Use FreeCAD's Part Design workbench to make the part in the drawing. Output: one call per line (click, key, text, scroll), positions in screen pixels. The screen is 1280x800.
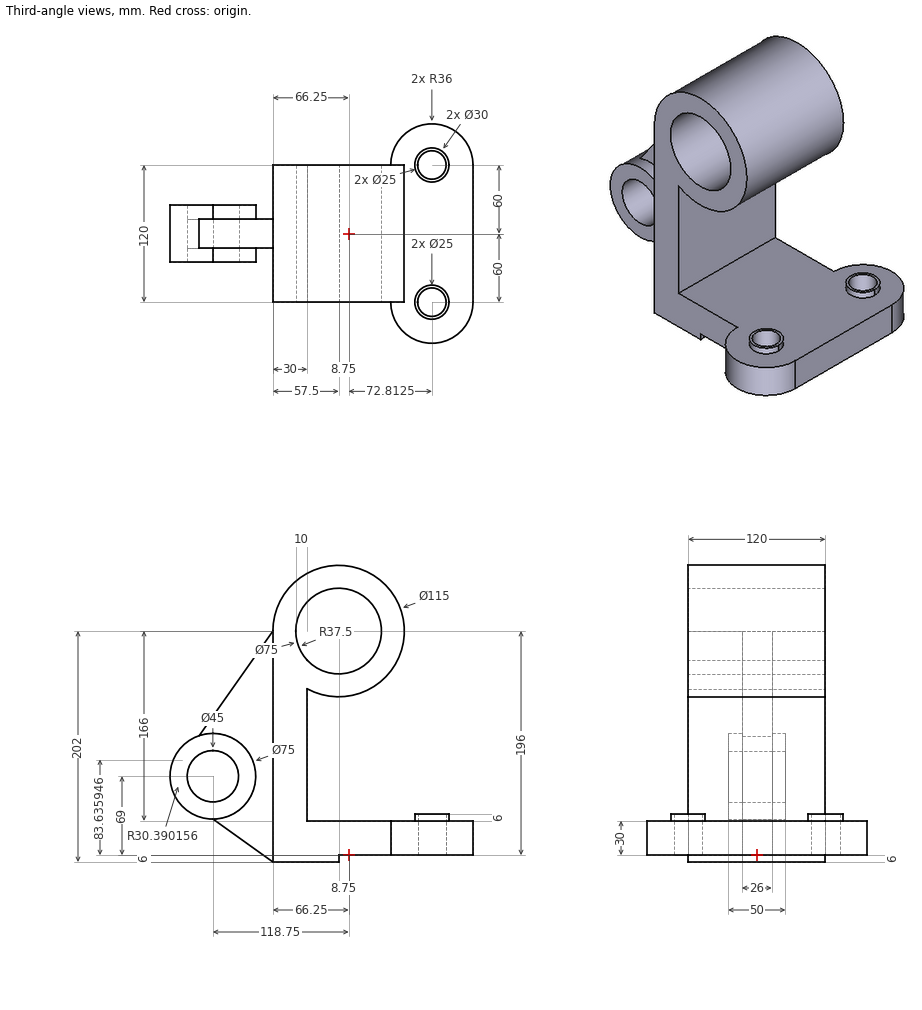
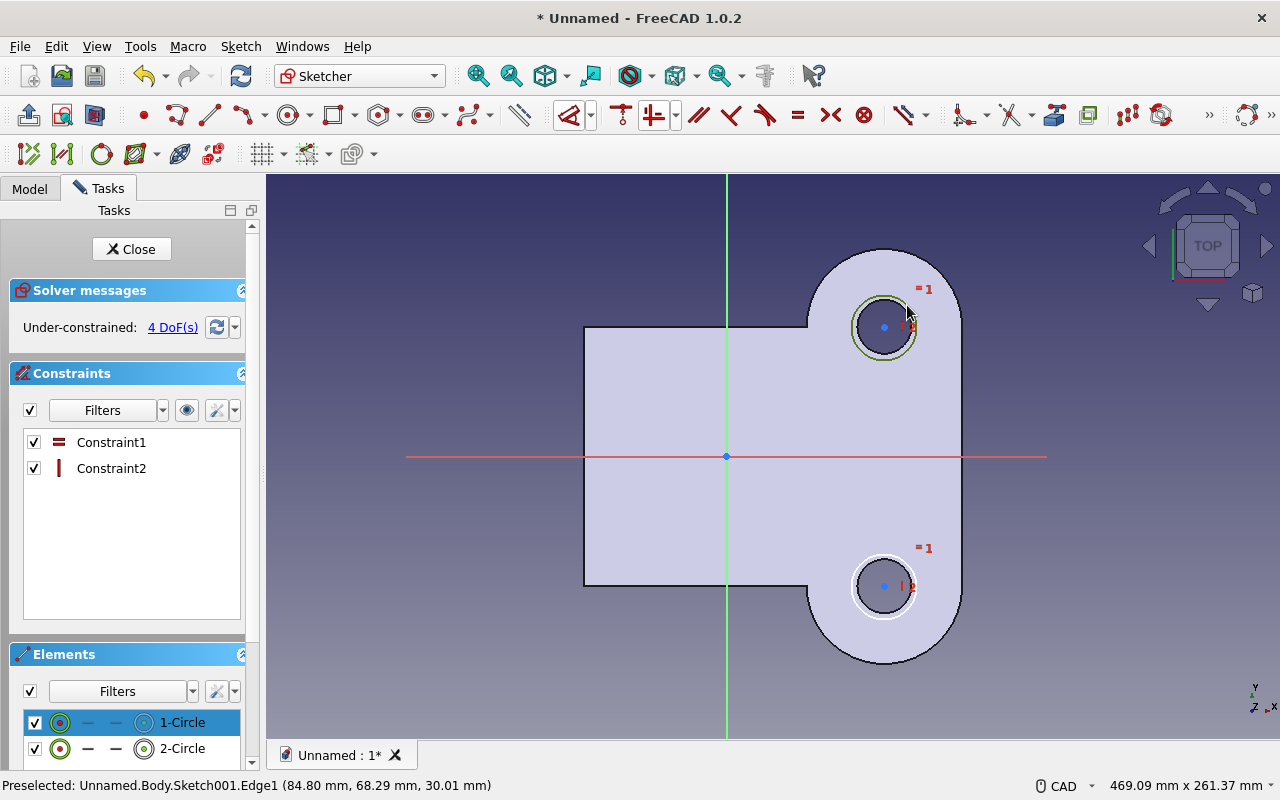
key(k)
key(o)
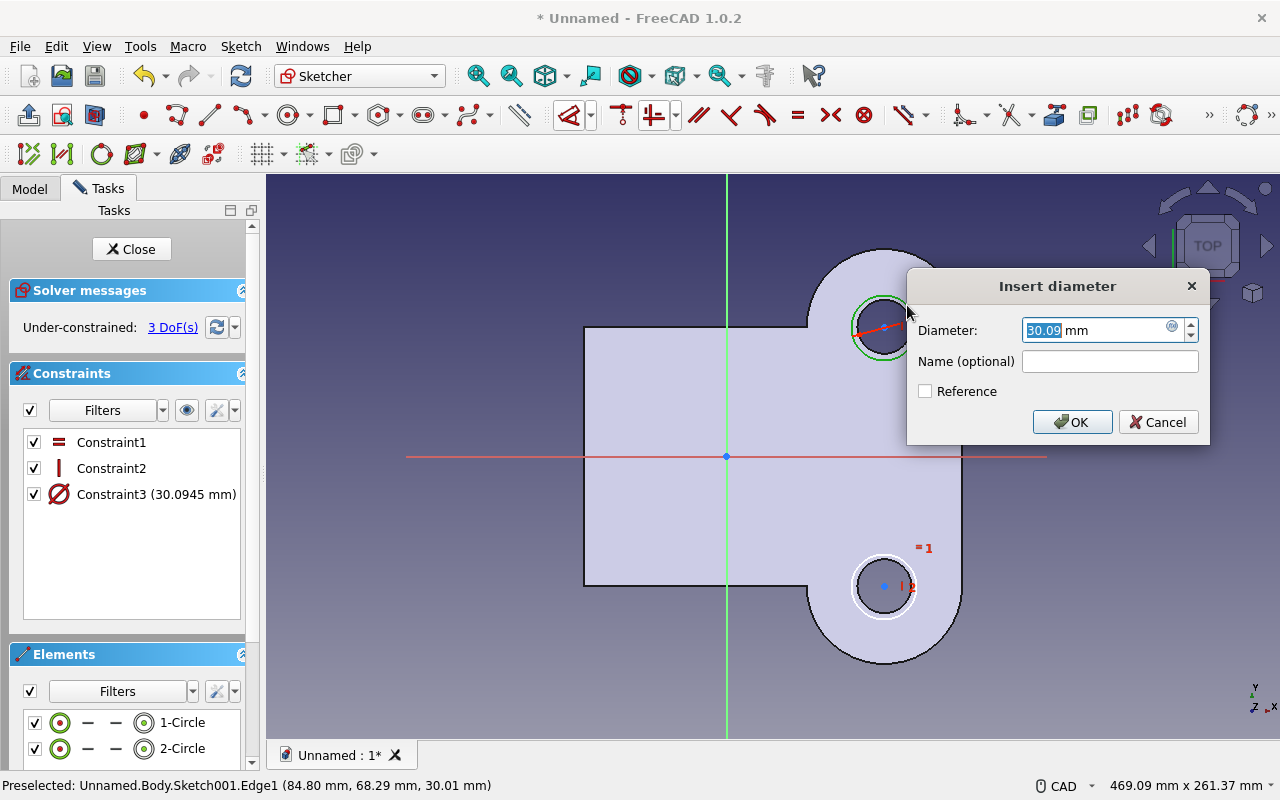
text(30)
key(Return)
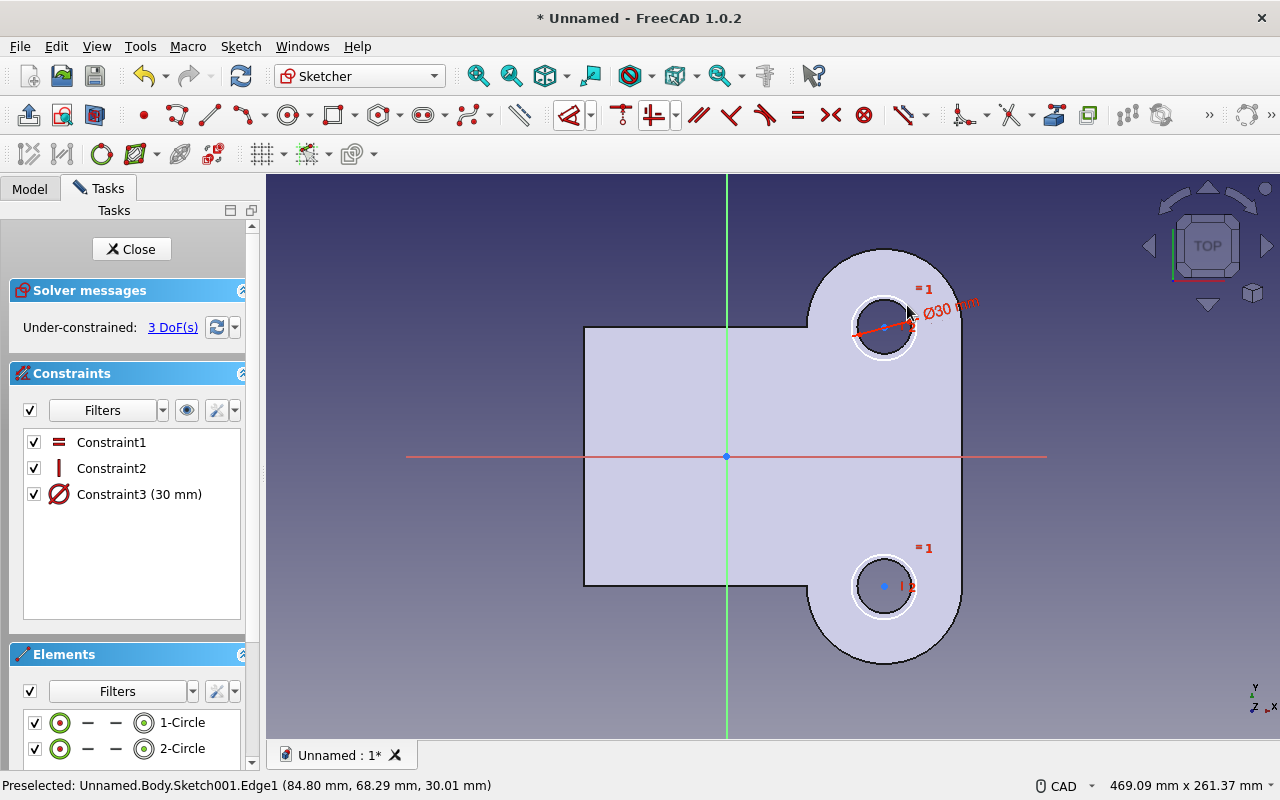
click(884, 328)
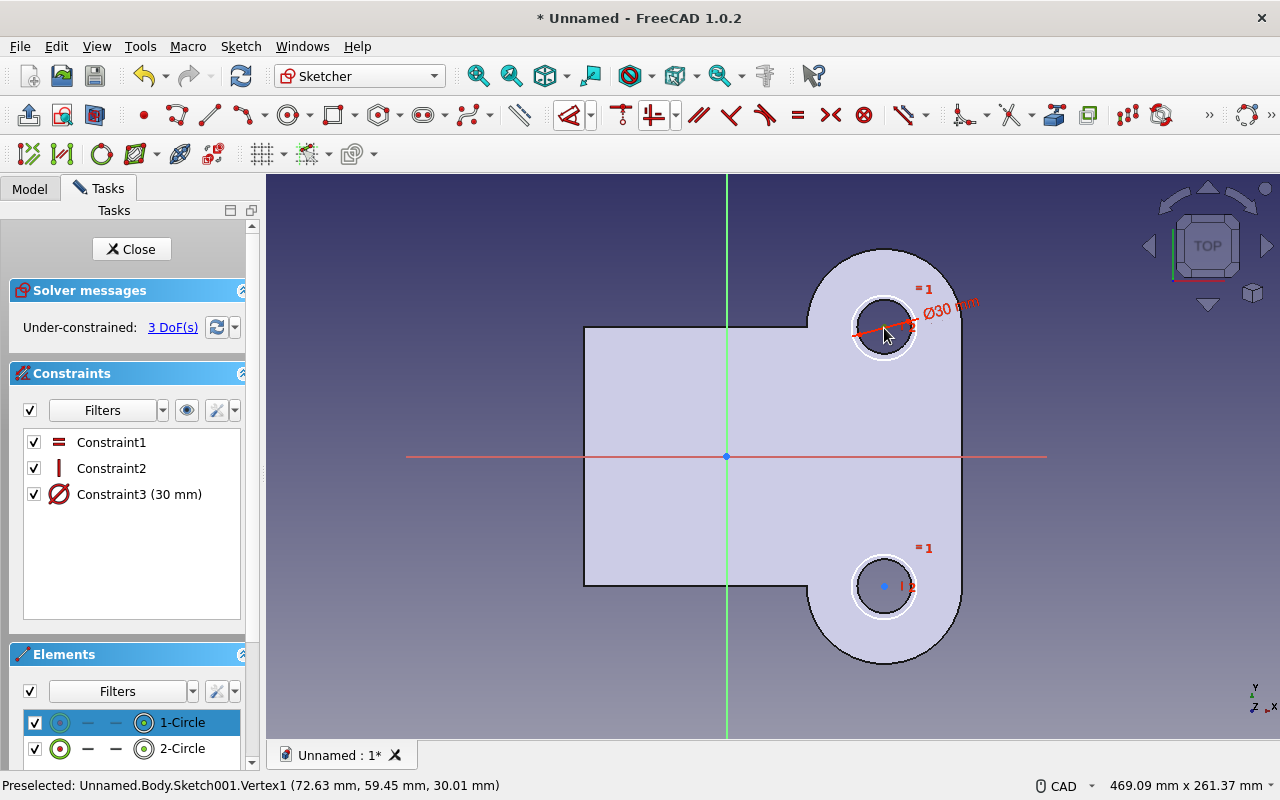
key(i)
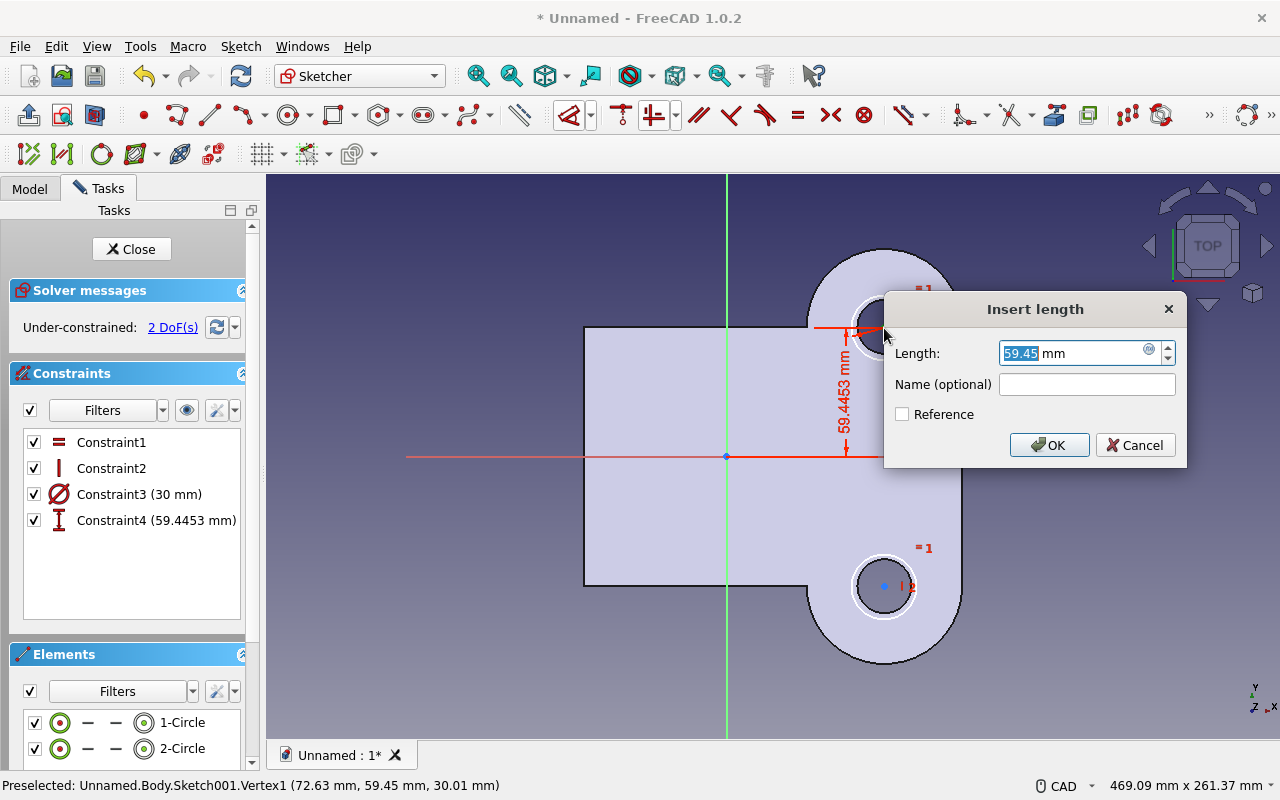
text(60)
key(Return)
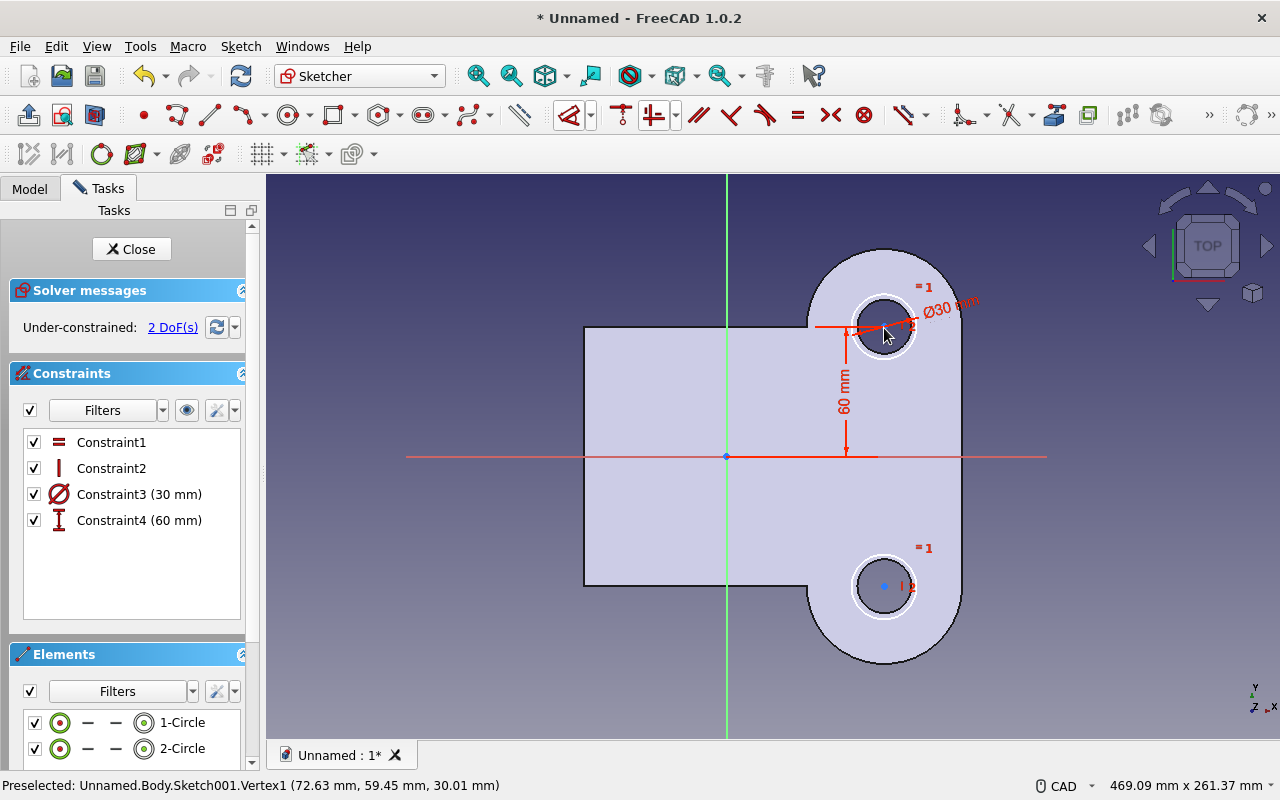
click(884, 587)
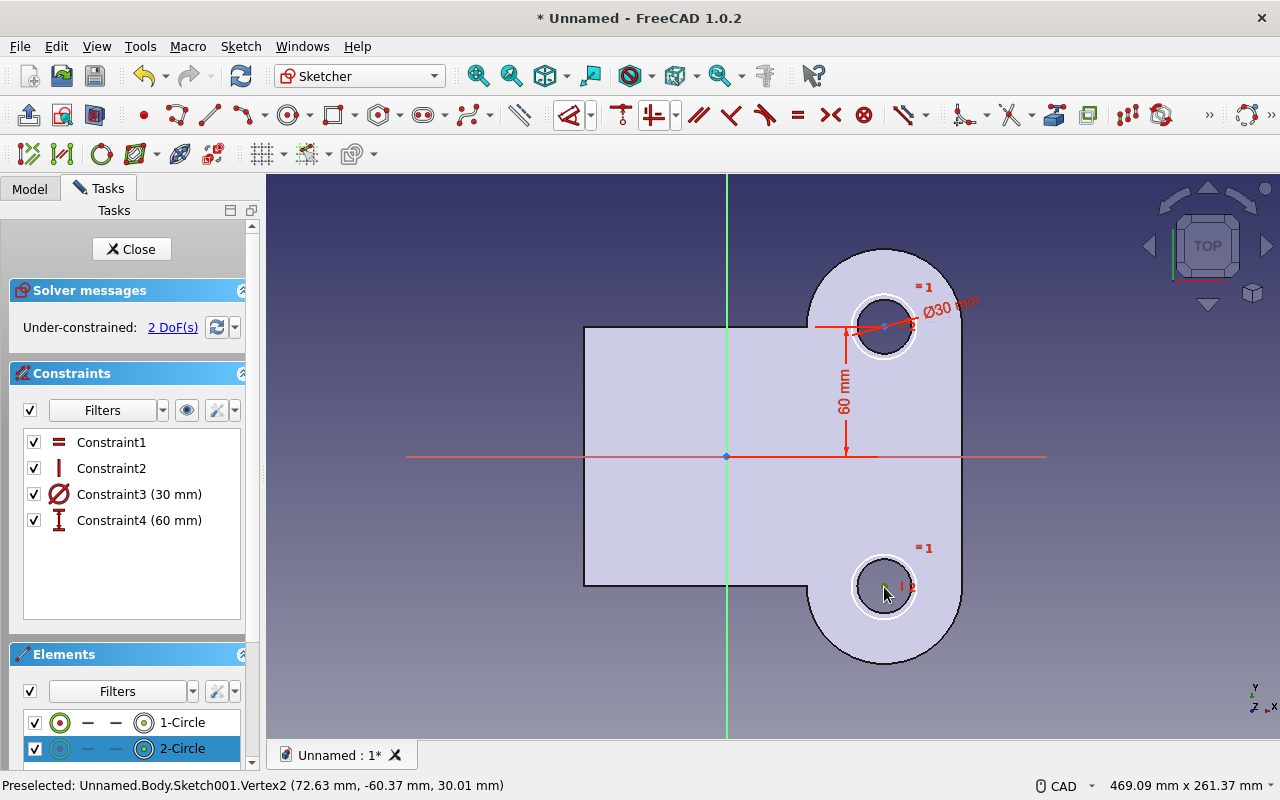
key(i)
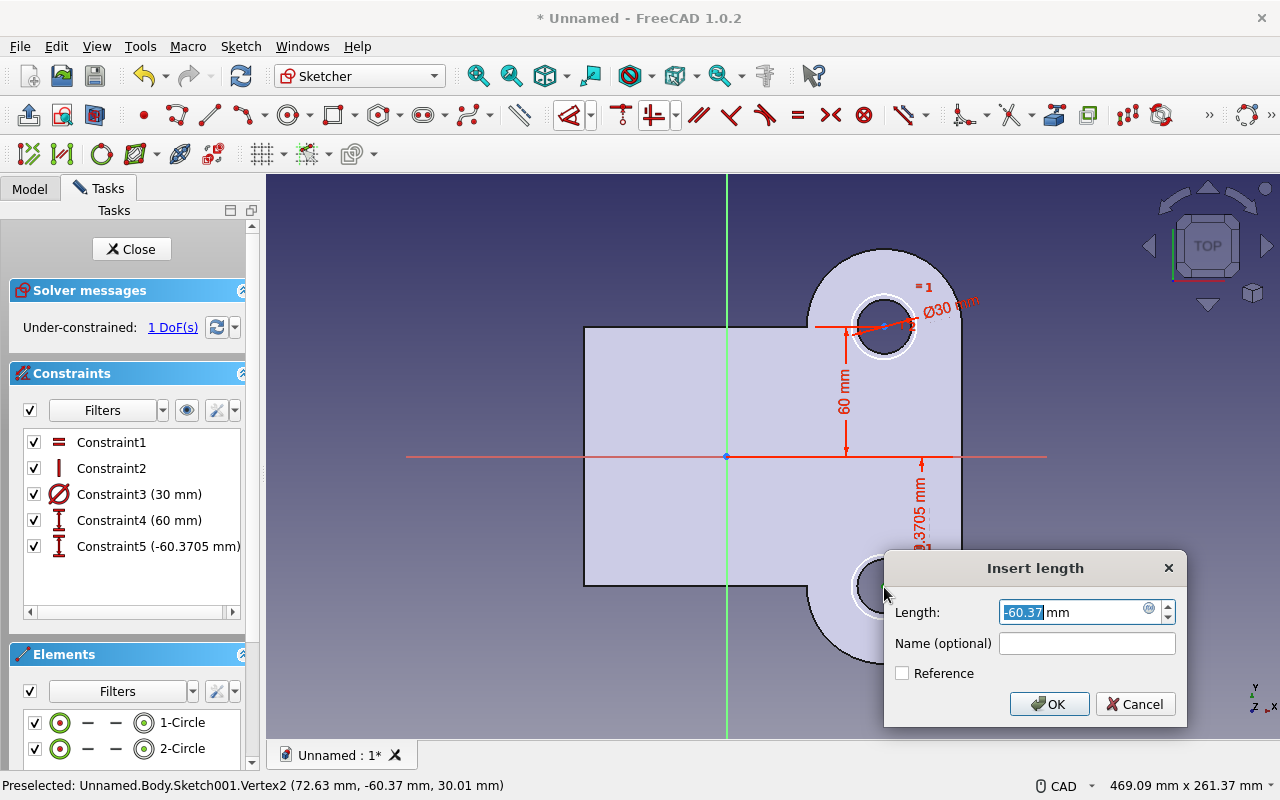
text(-60)
key(Return)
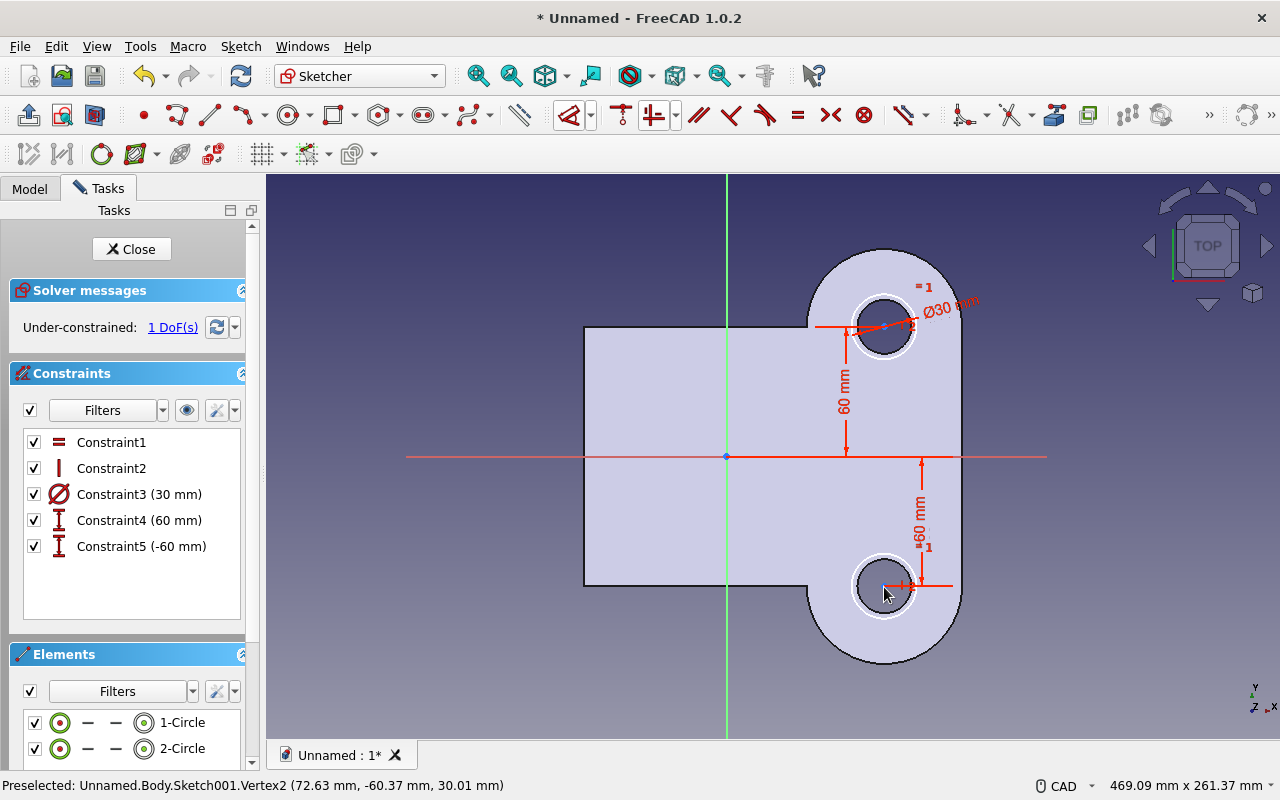
click(884, 327)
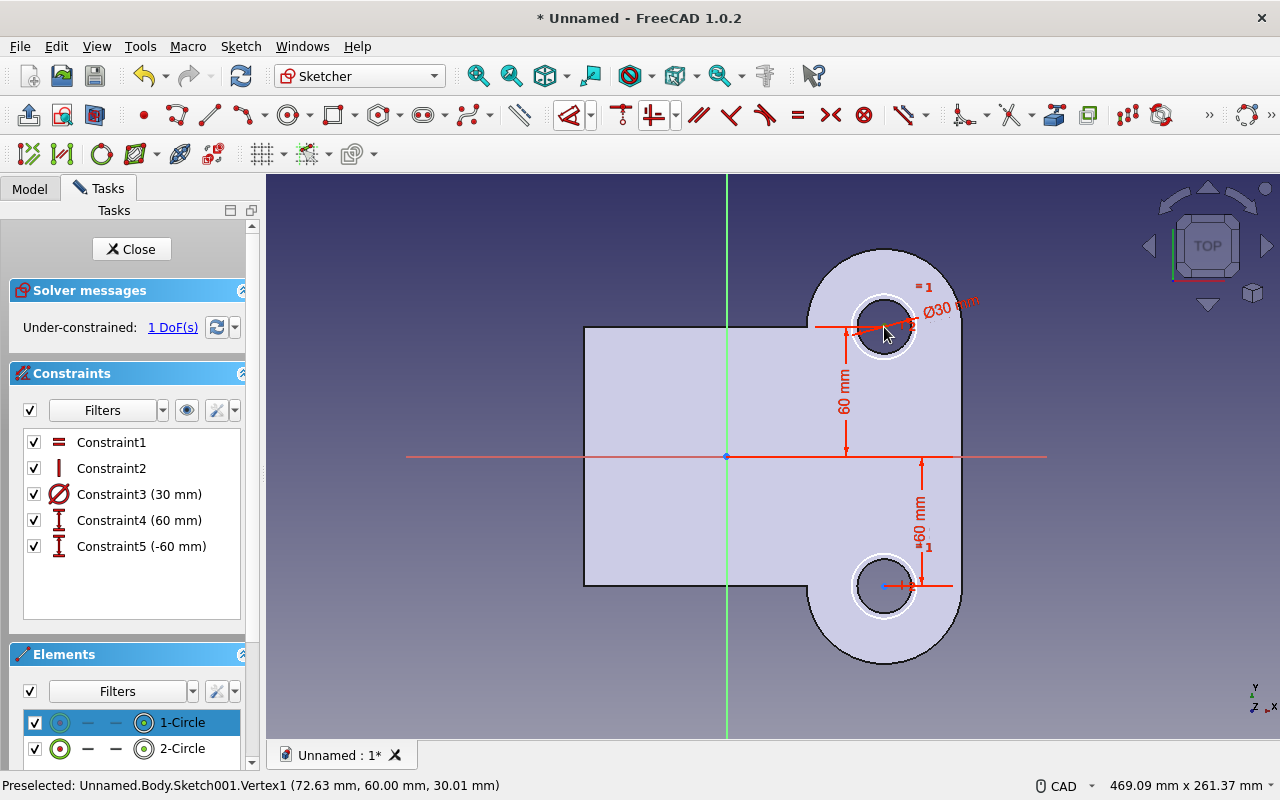
key(l)